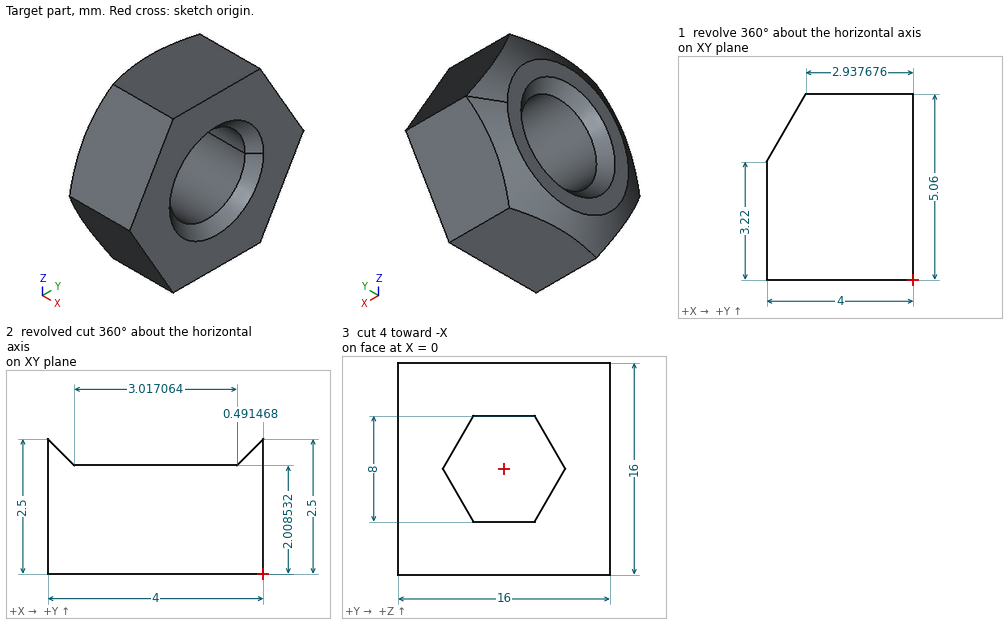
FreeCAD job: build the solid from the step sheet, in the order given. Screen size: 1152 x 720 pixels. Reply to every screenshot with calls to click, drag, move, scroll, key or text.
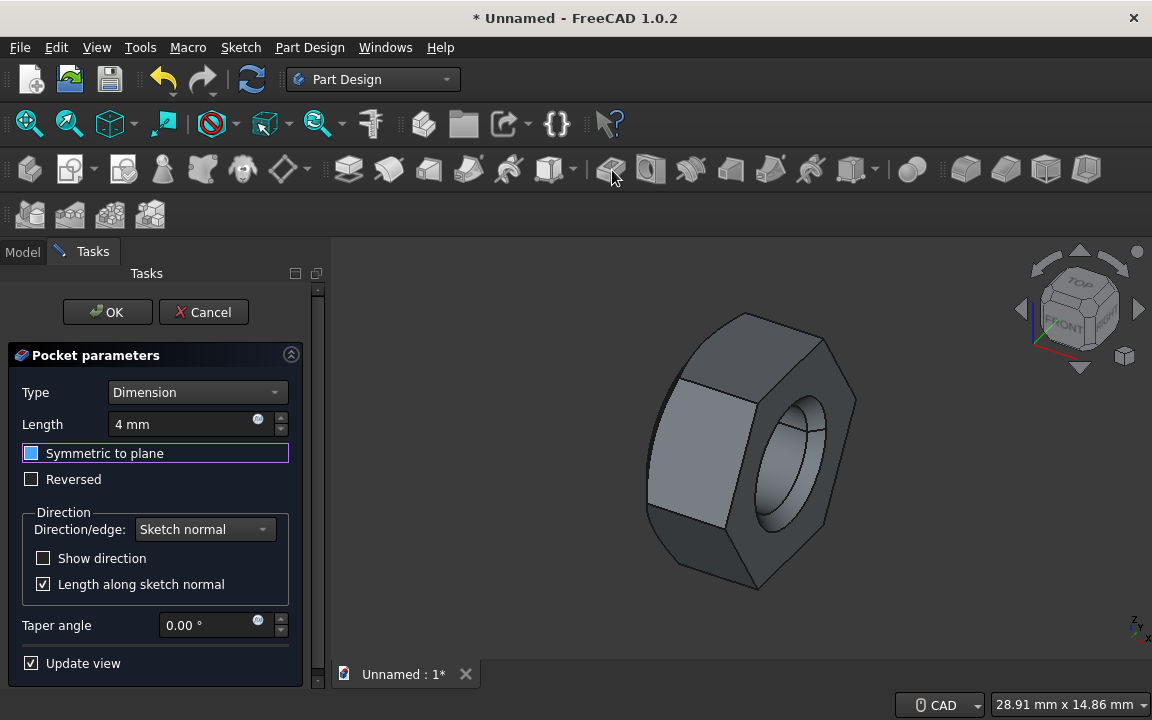
click(108, 312)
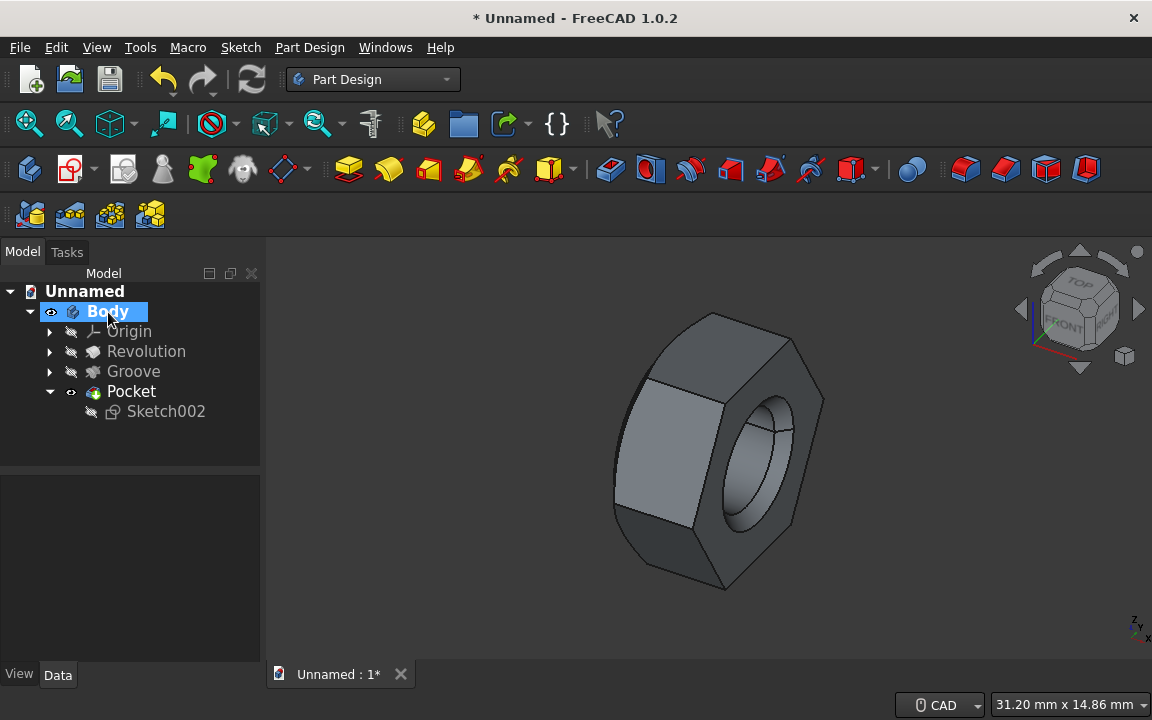
key(0)